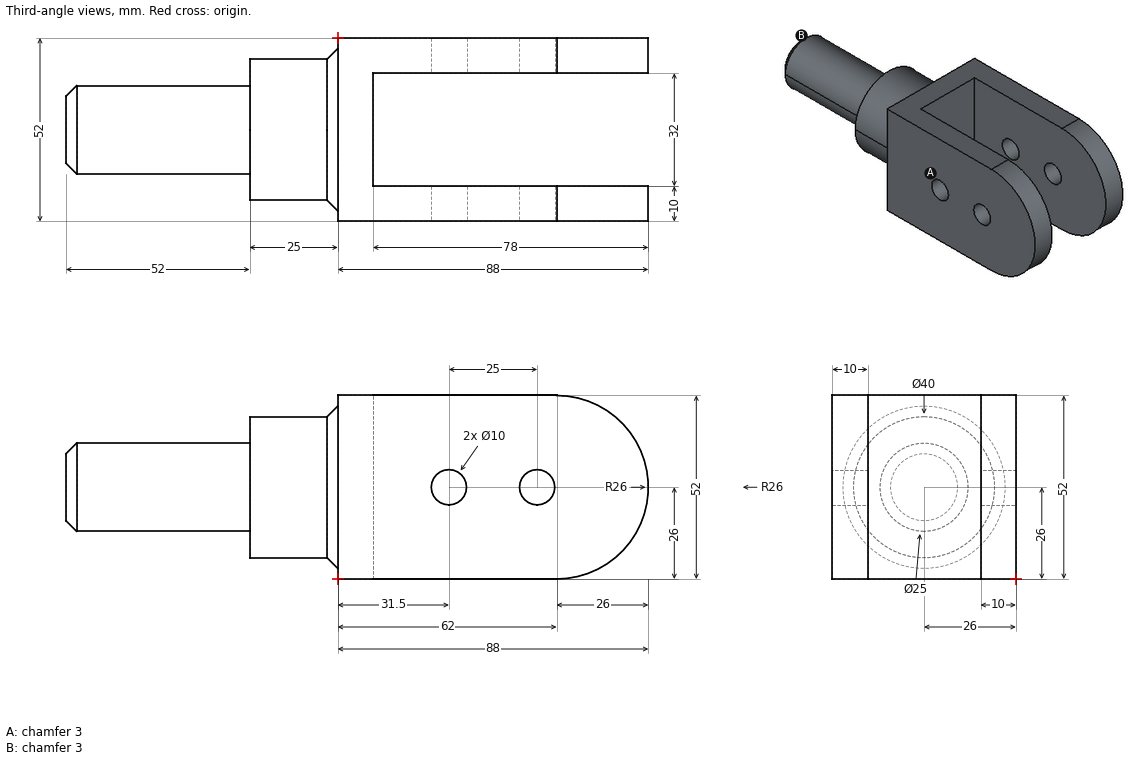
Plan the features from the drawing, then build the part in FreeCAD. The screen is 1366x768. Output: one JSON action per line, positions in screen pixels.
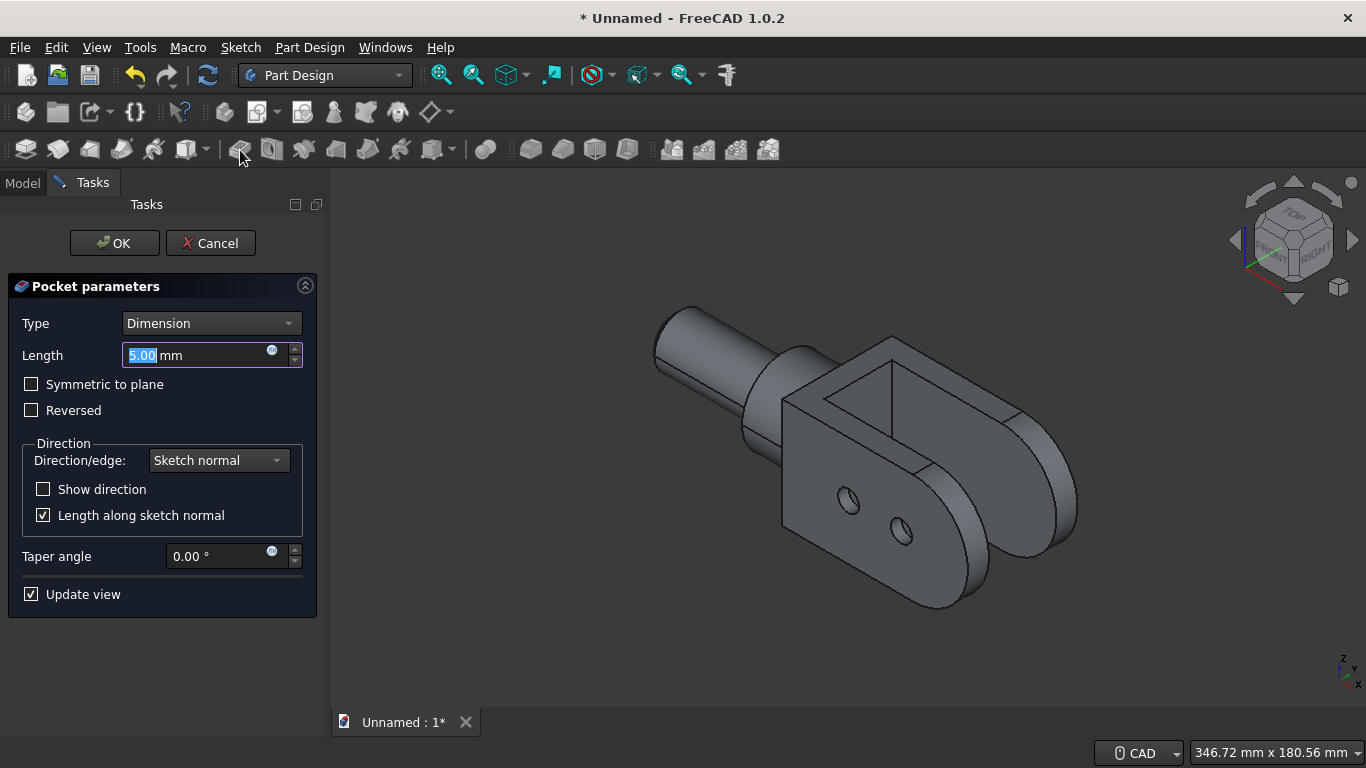
{"action": "type", "text": "52"}
{"action": "key", "text": "Tab"}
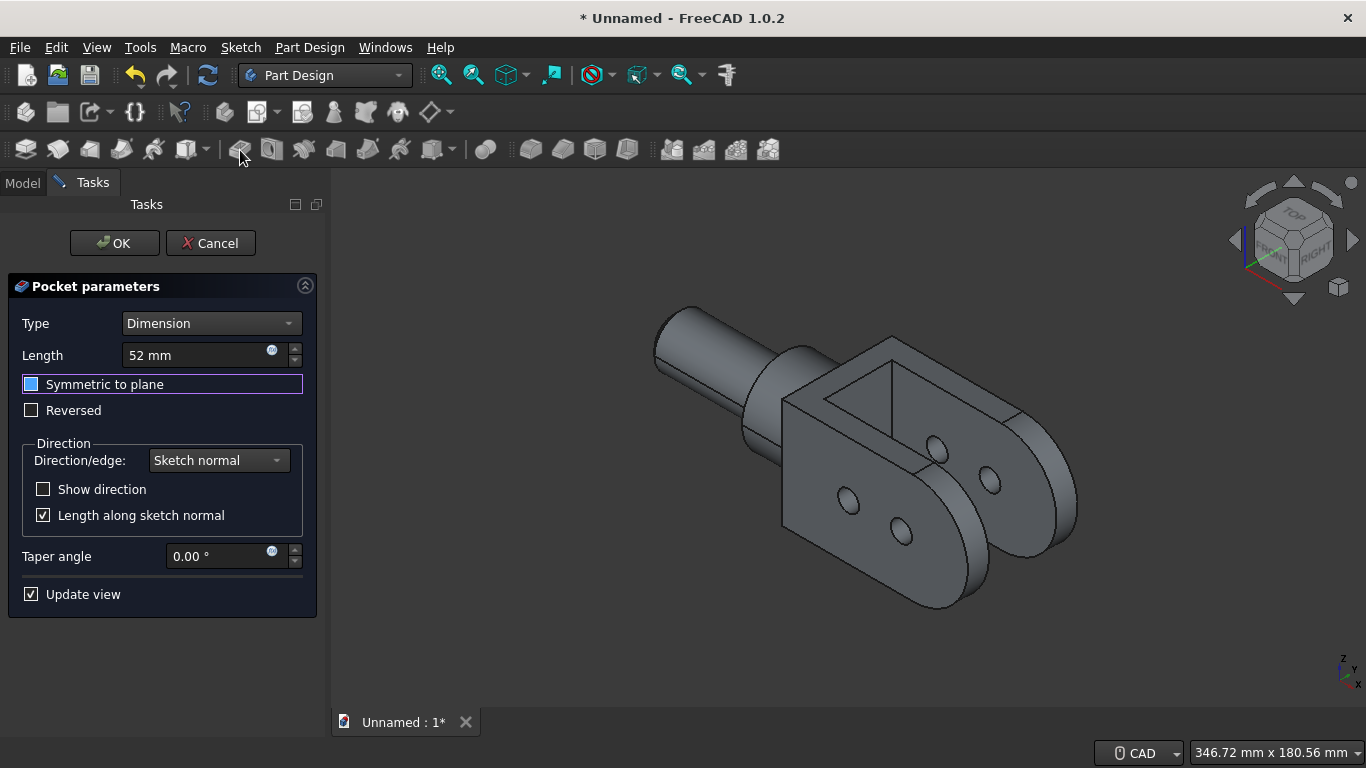
{"action": "left_click", "coordinate": [115, 243]}